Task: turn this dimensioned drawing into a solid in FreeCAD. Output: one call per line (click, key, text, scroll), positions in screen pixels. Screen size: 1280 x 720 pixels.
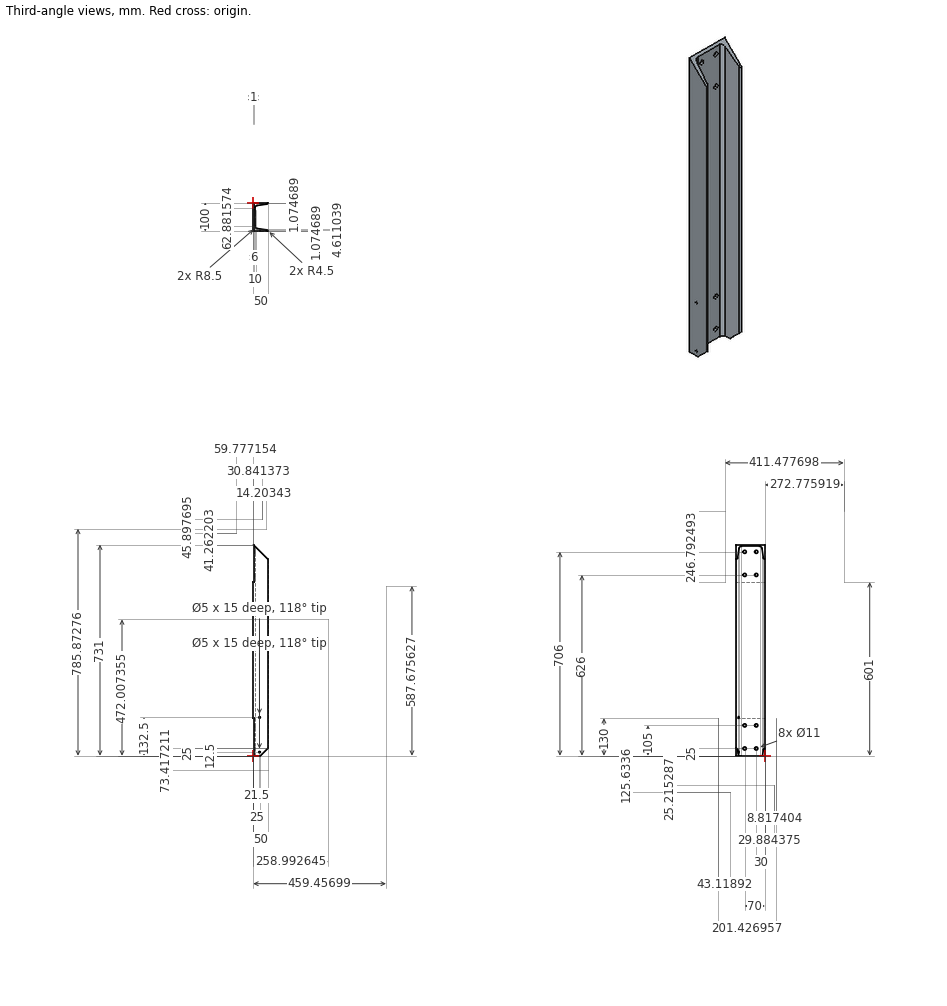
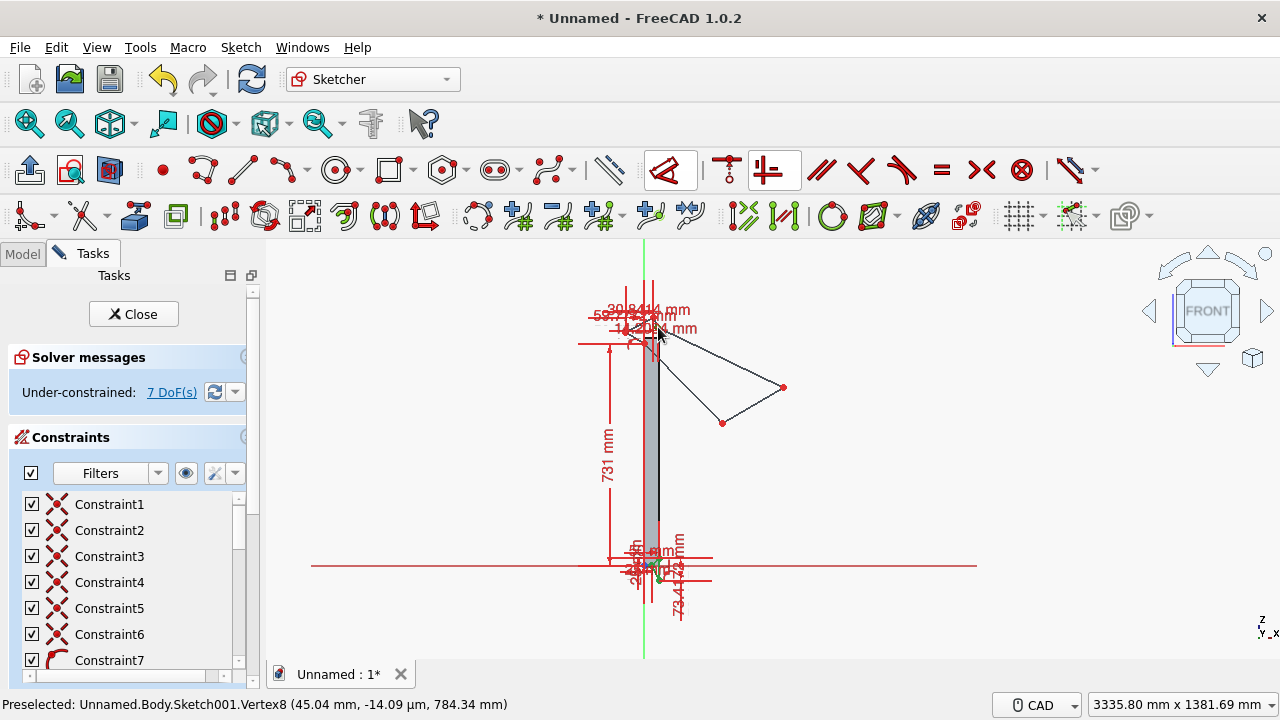
key(i)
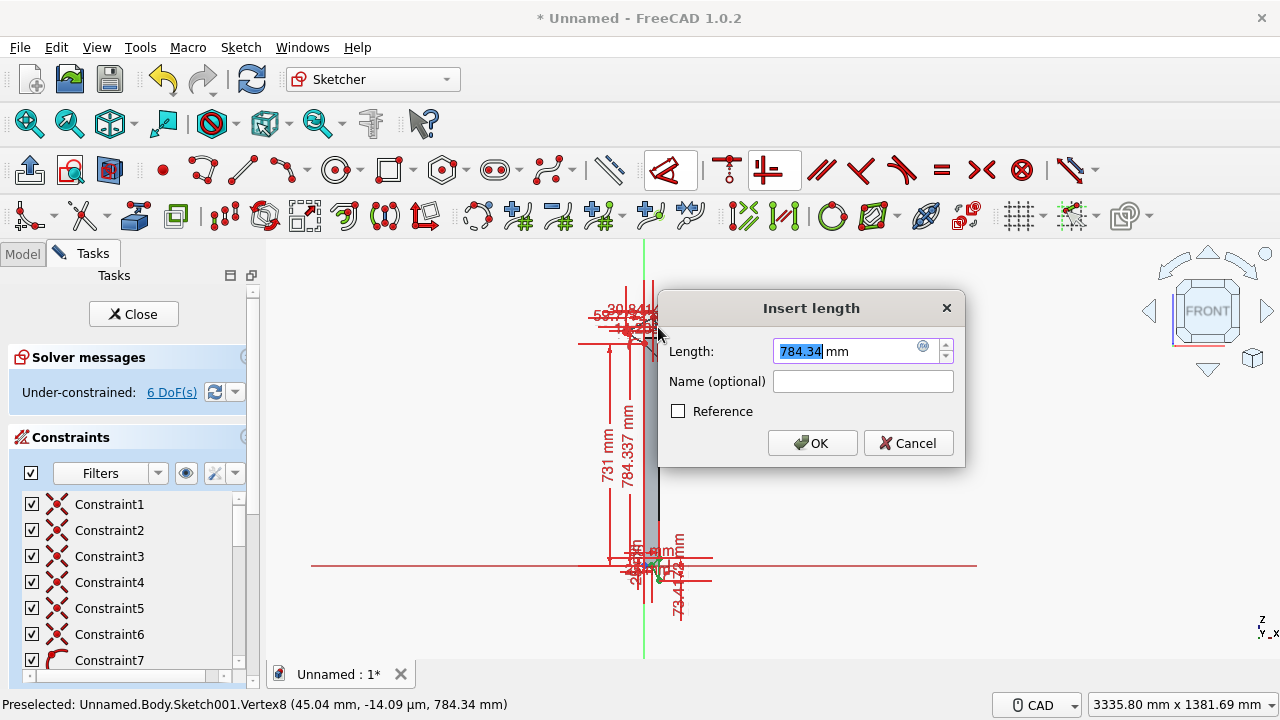
text(785.87276)
key(Return)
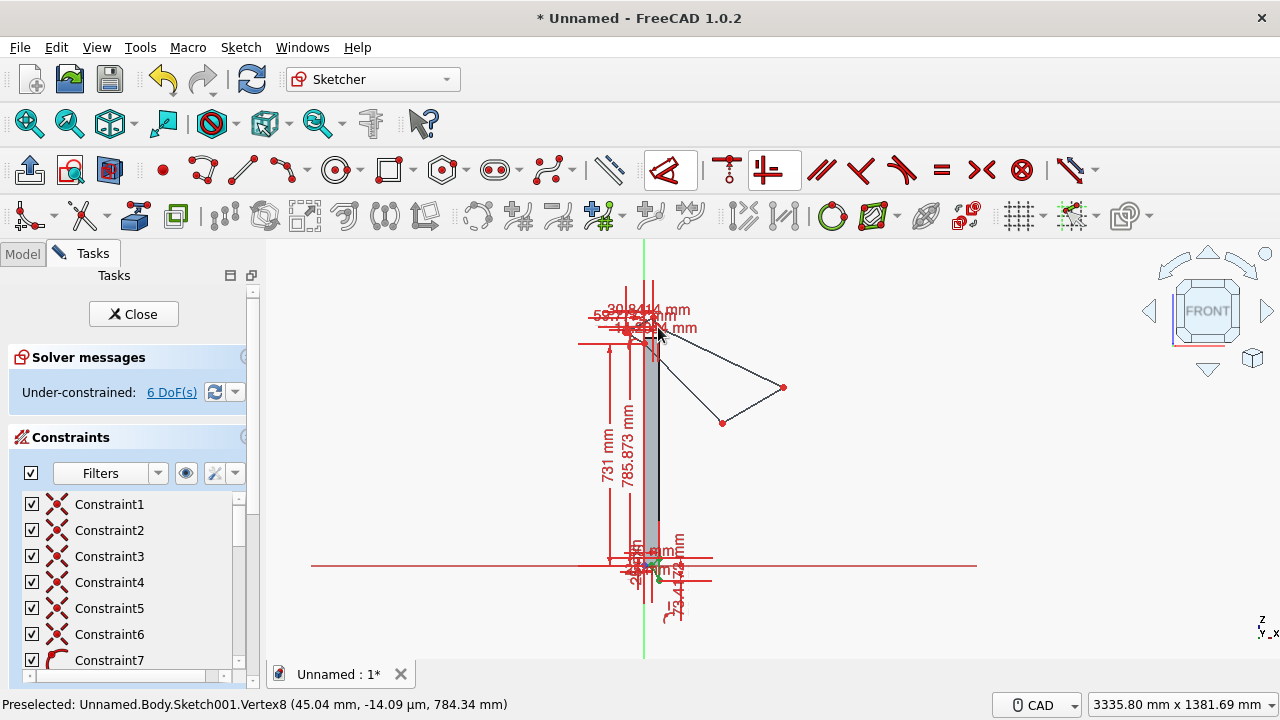
click(784, 388)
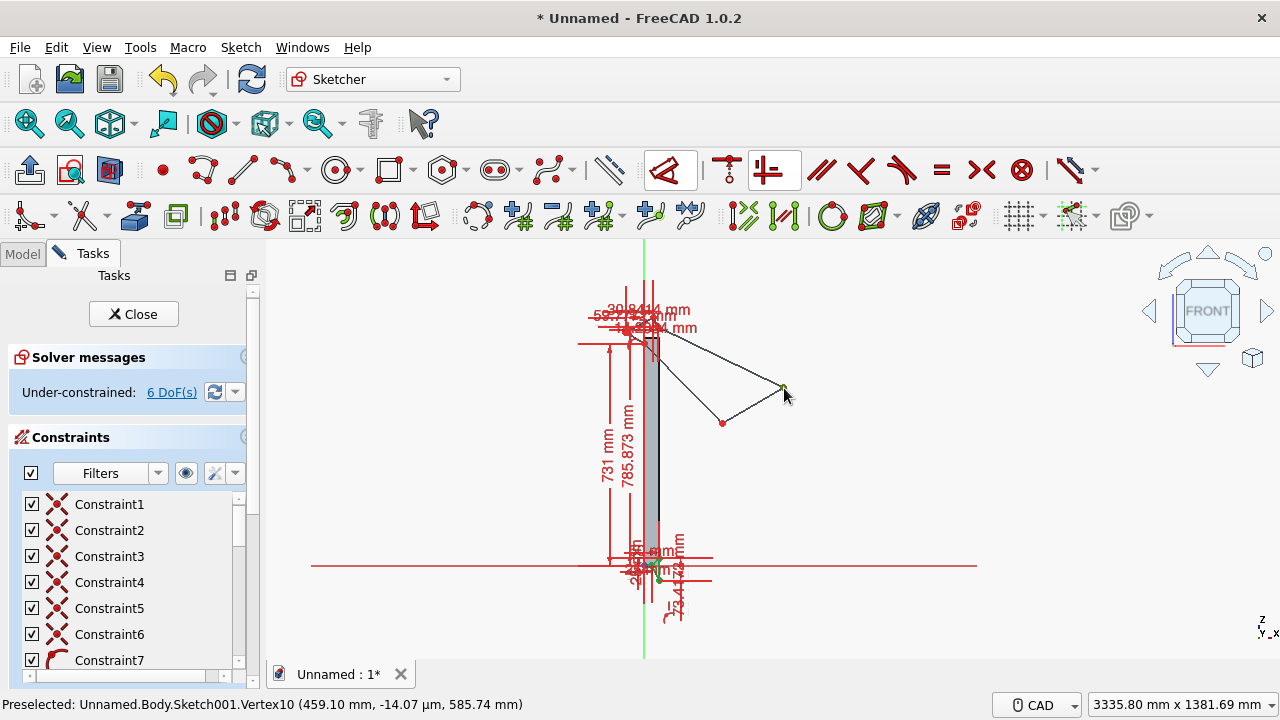
key(l)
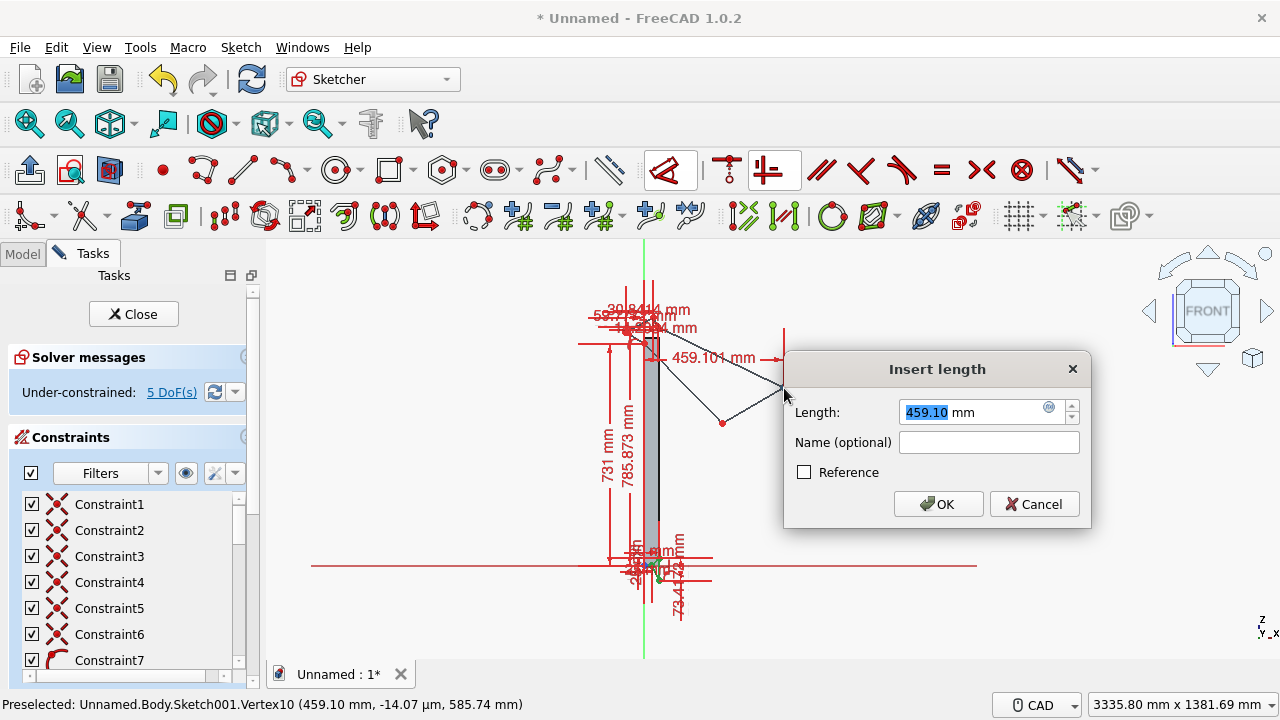
text(459.45699)
key(Return)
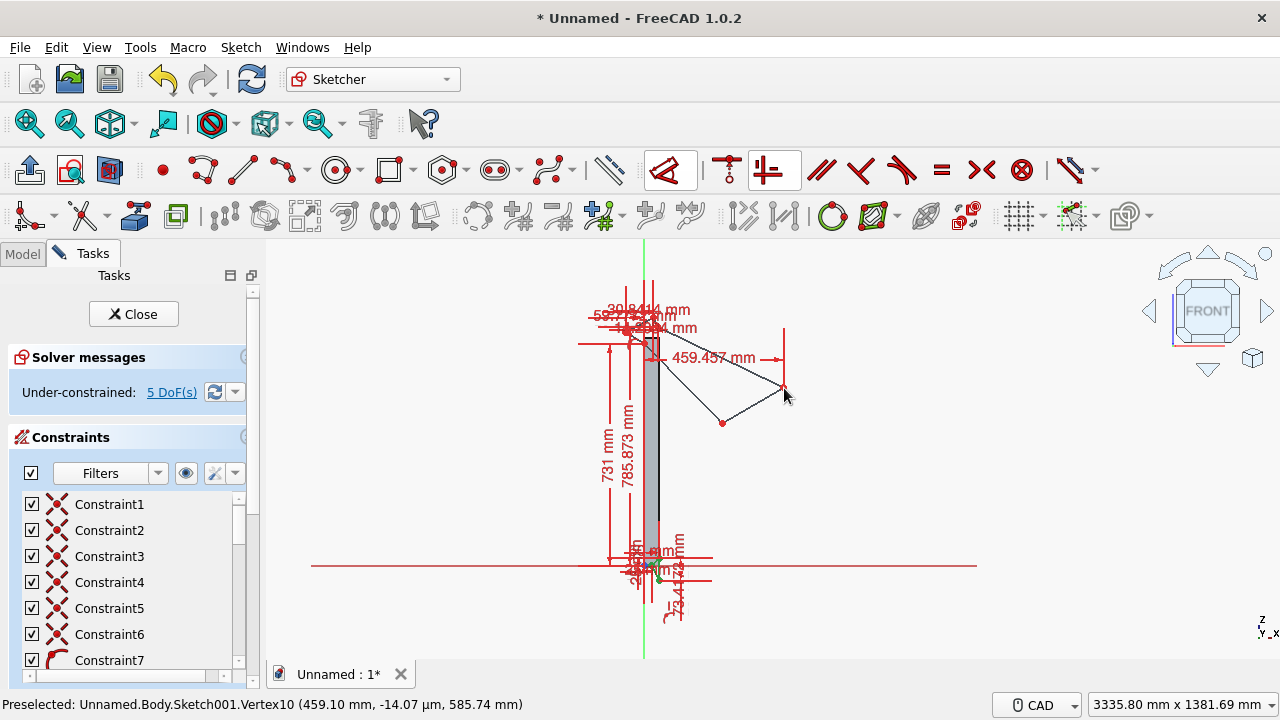
scroll(635, 338, up, 6)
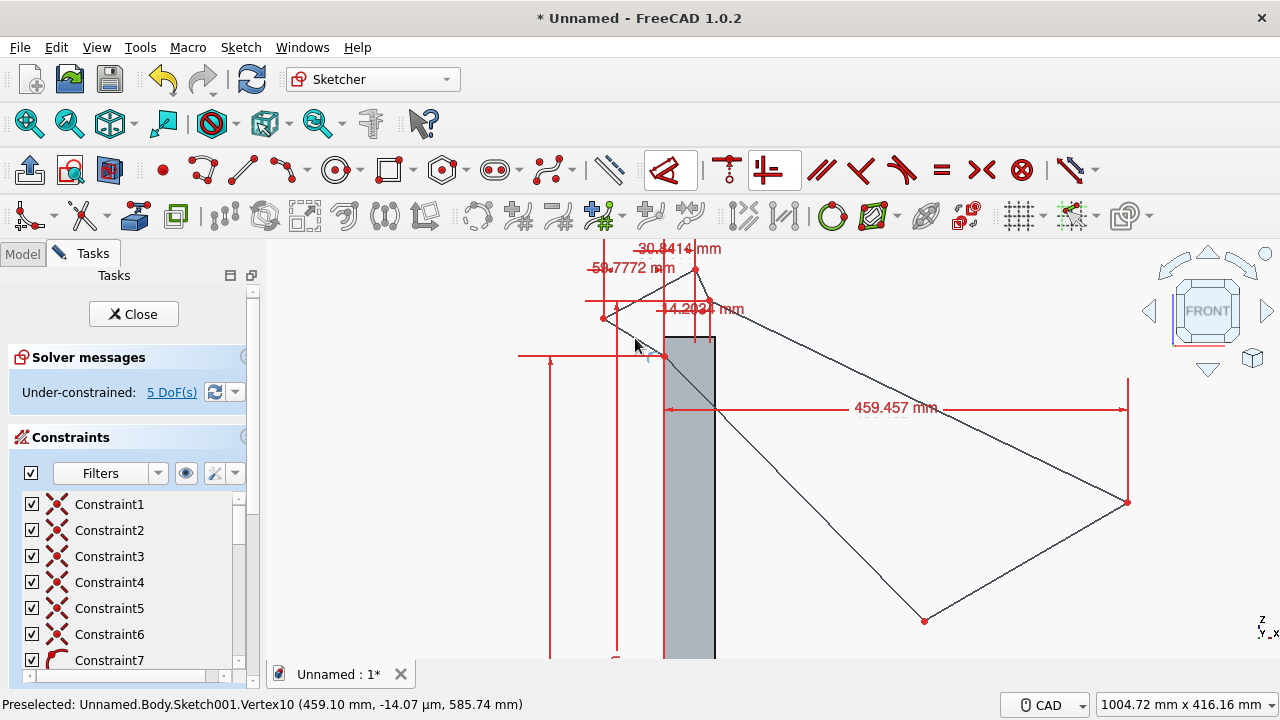
click(634, 337)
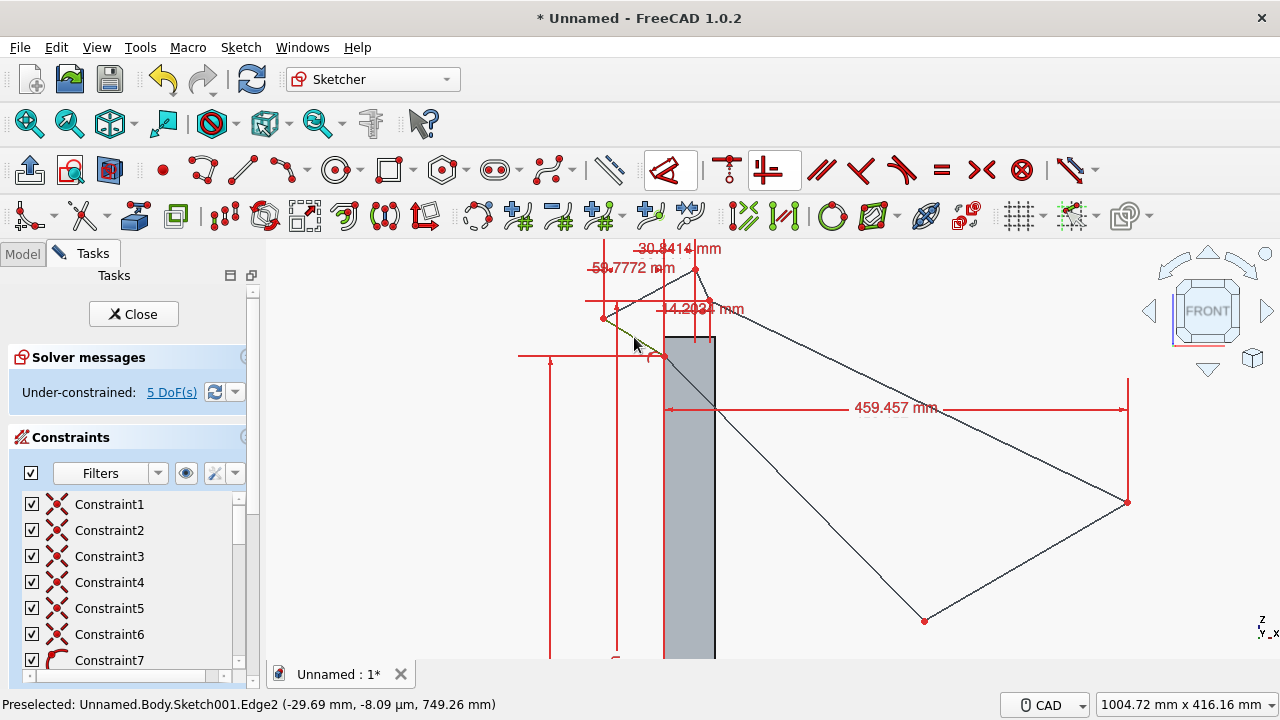
click(692, 170)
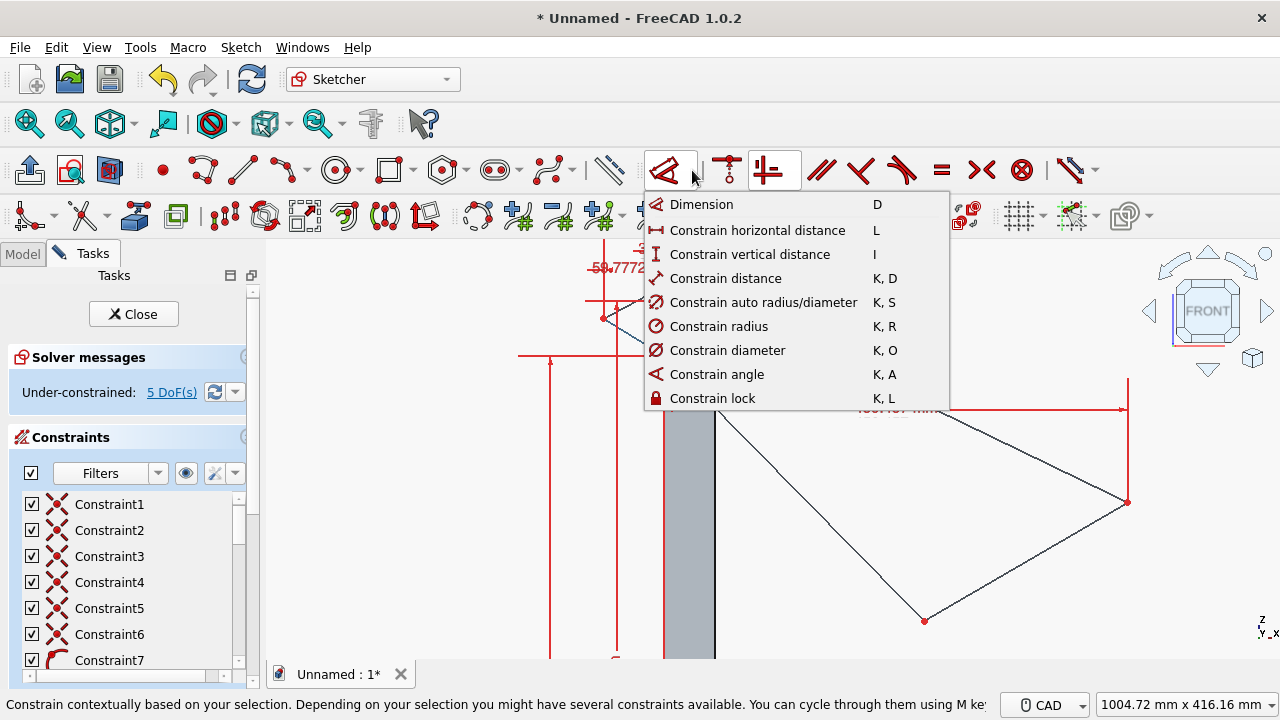
click(797, 254)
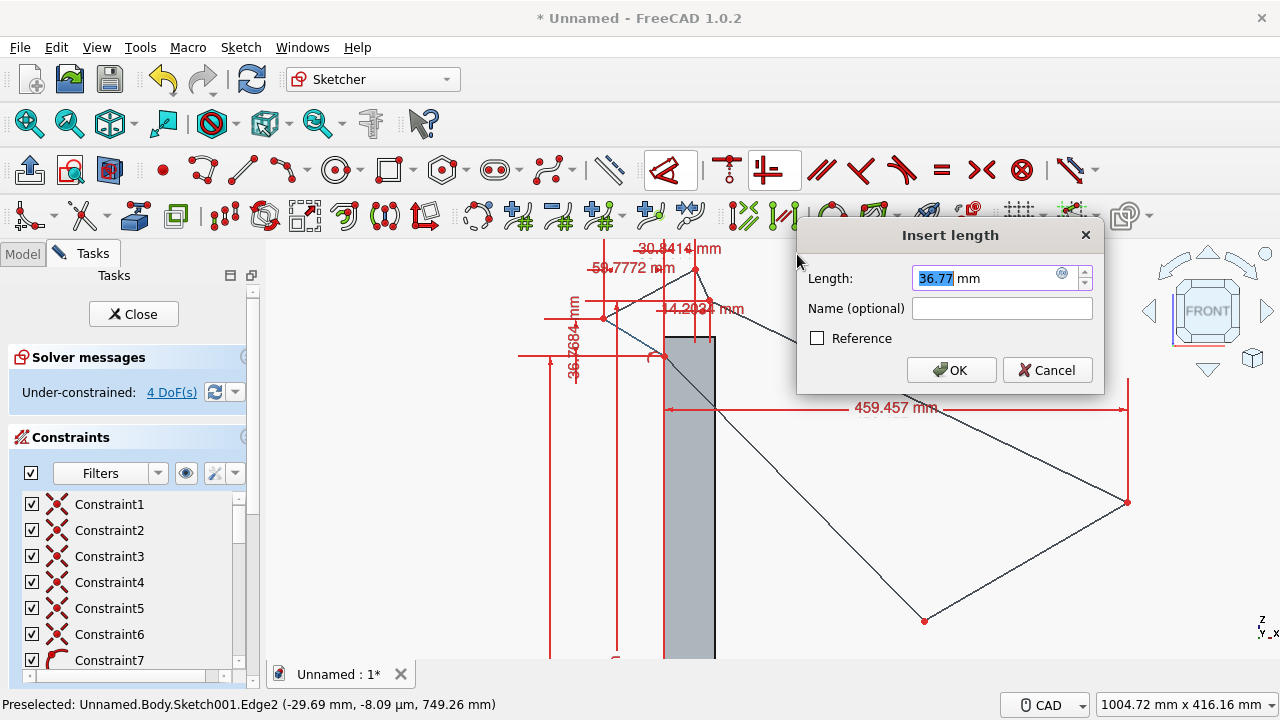
text(41.262203)
key(Return)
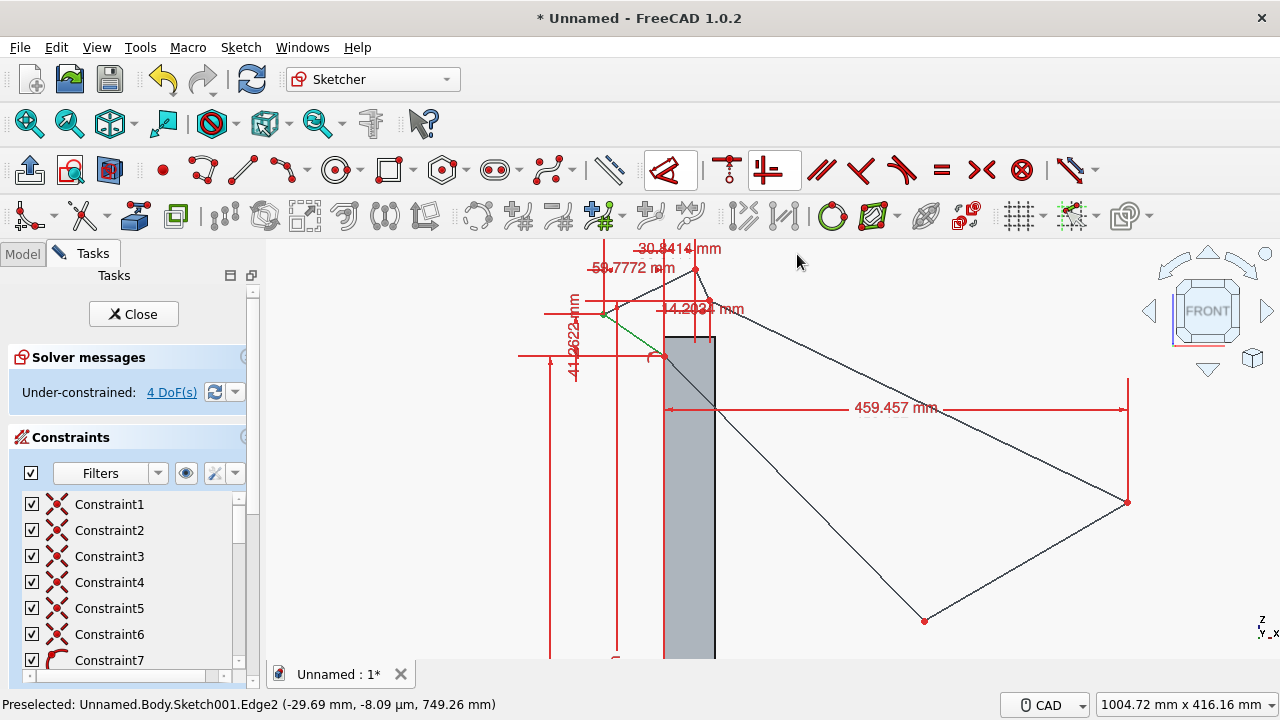
click(631, 301)